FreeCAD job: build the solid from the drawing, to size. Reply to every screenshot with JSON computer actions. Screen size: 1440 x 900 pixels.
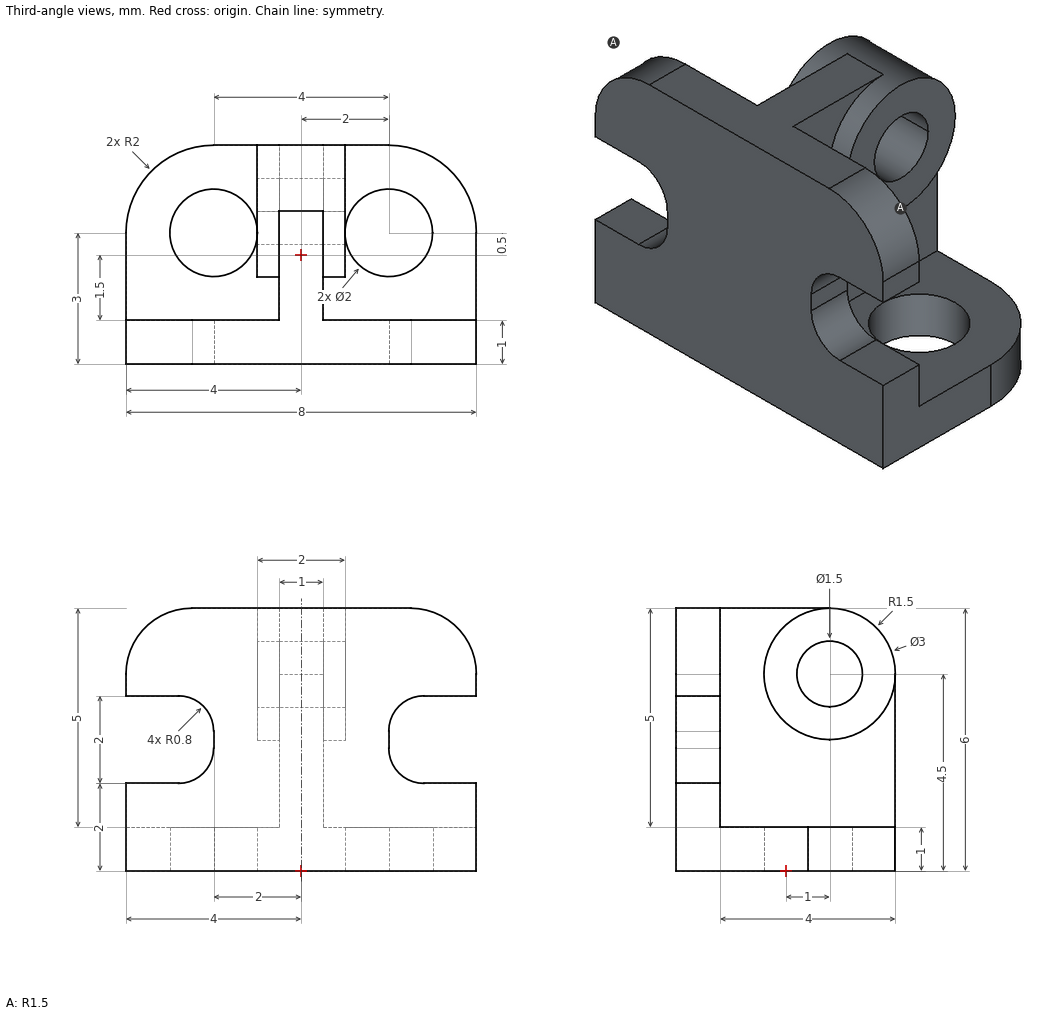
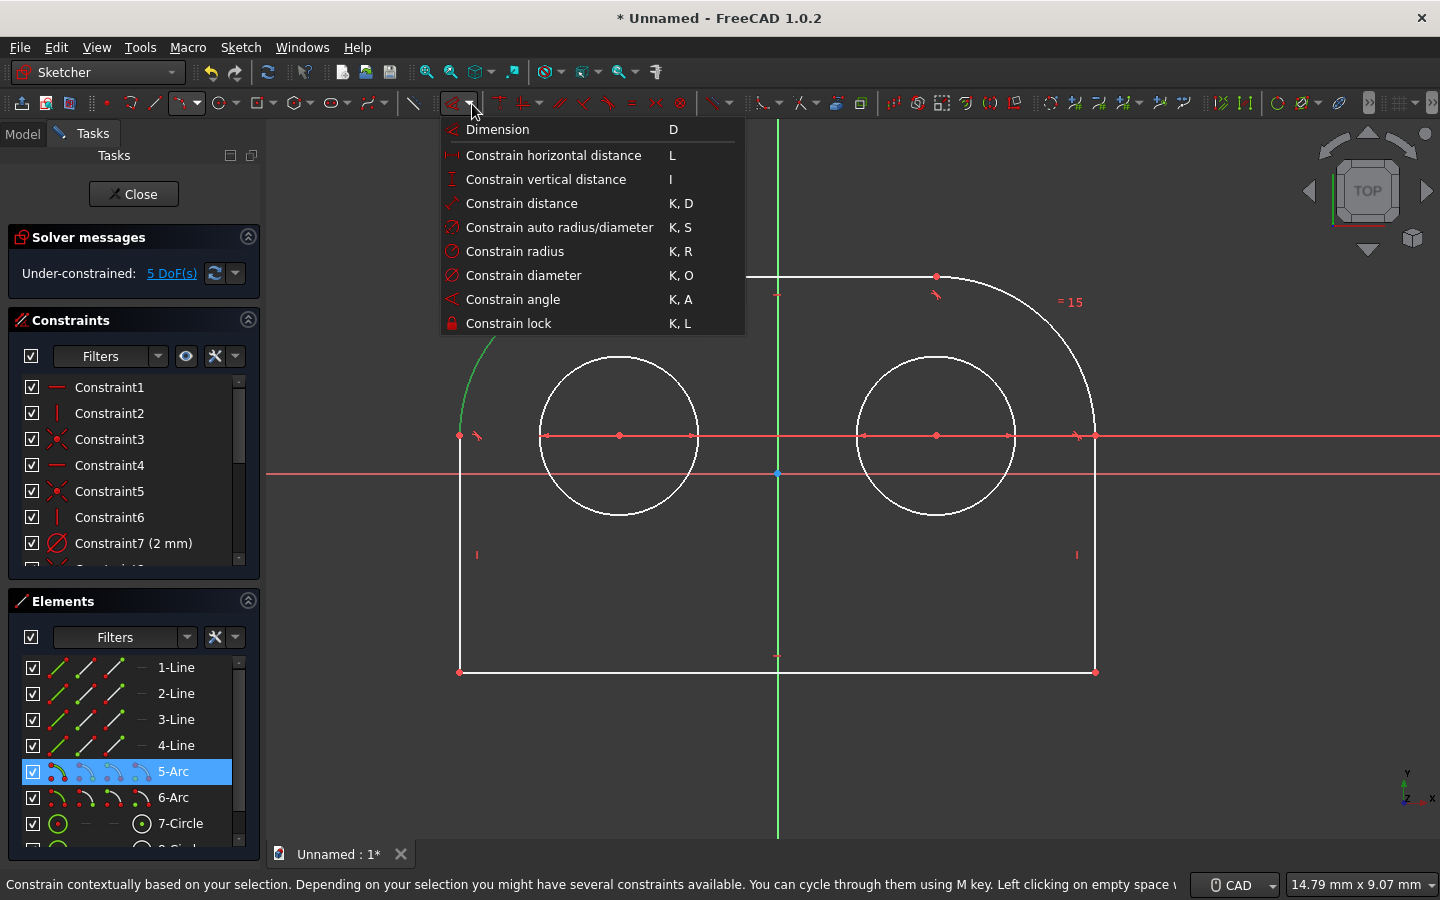
{"action": "left_click", "coordinate": [593, 251]}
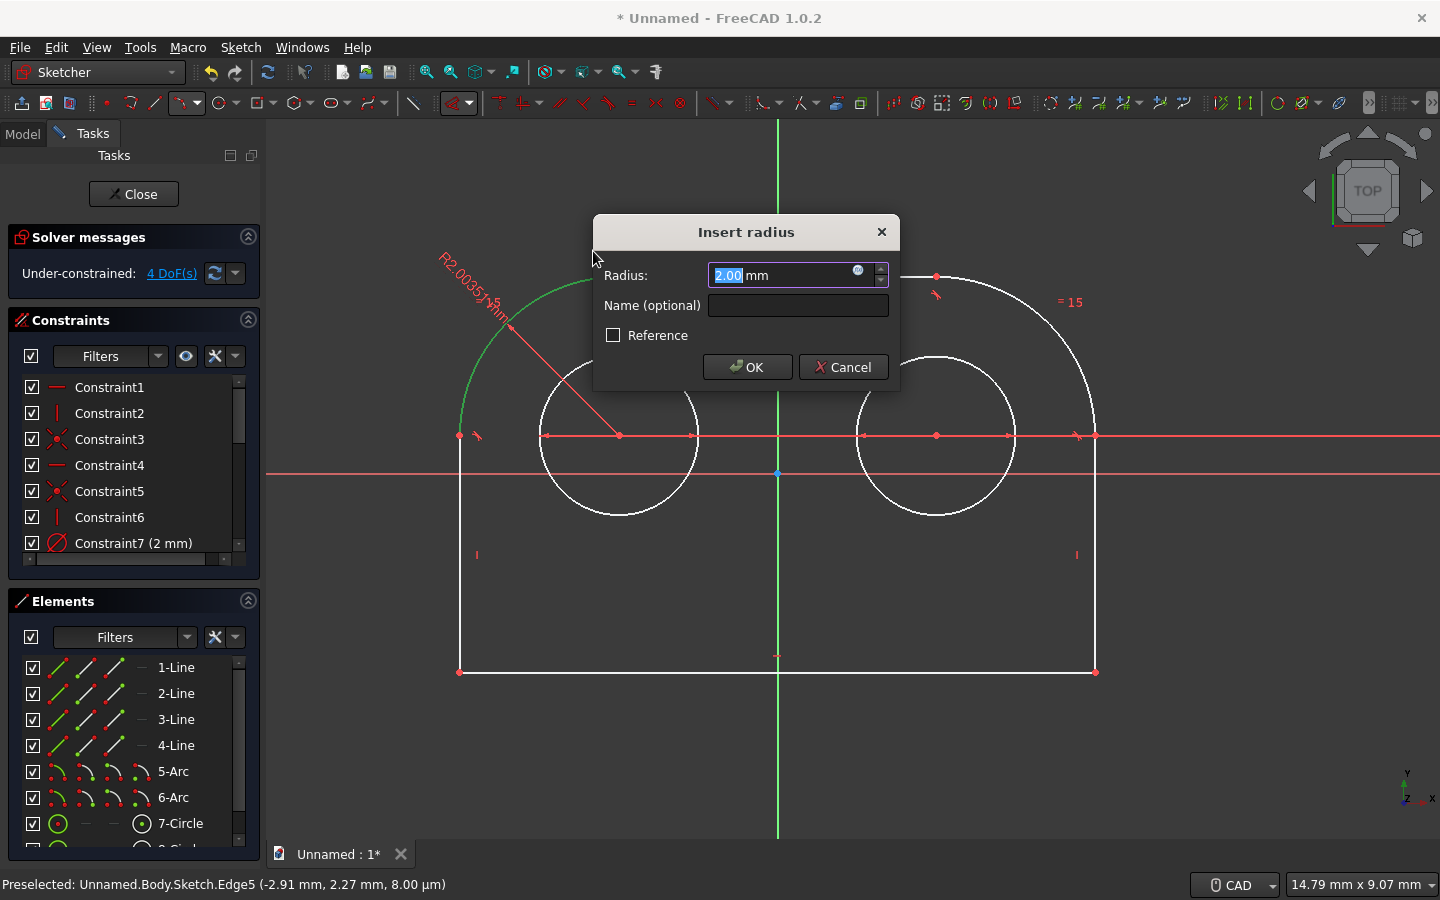
{"action": "type", "text": "2"}
{"action": "key", "text": "Return"}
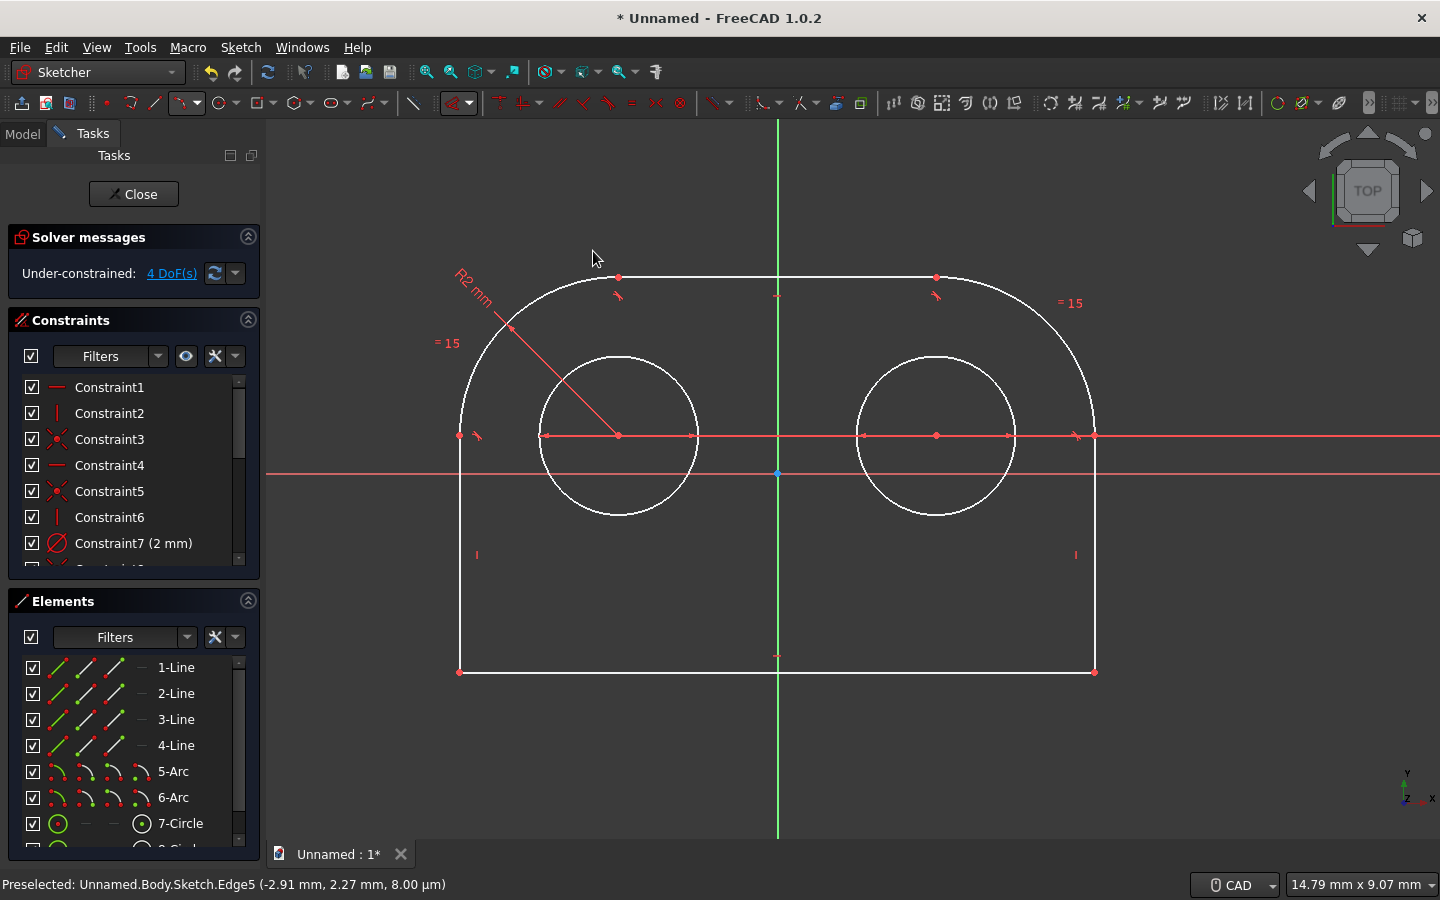
{"action": "left_click", "coordinate": [841, 277]}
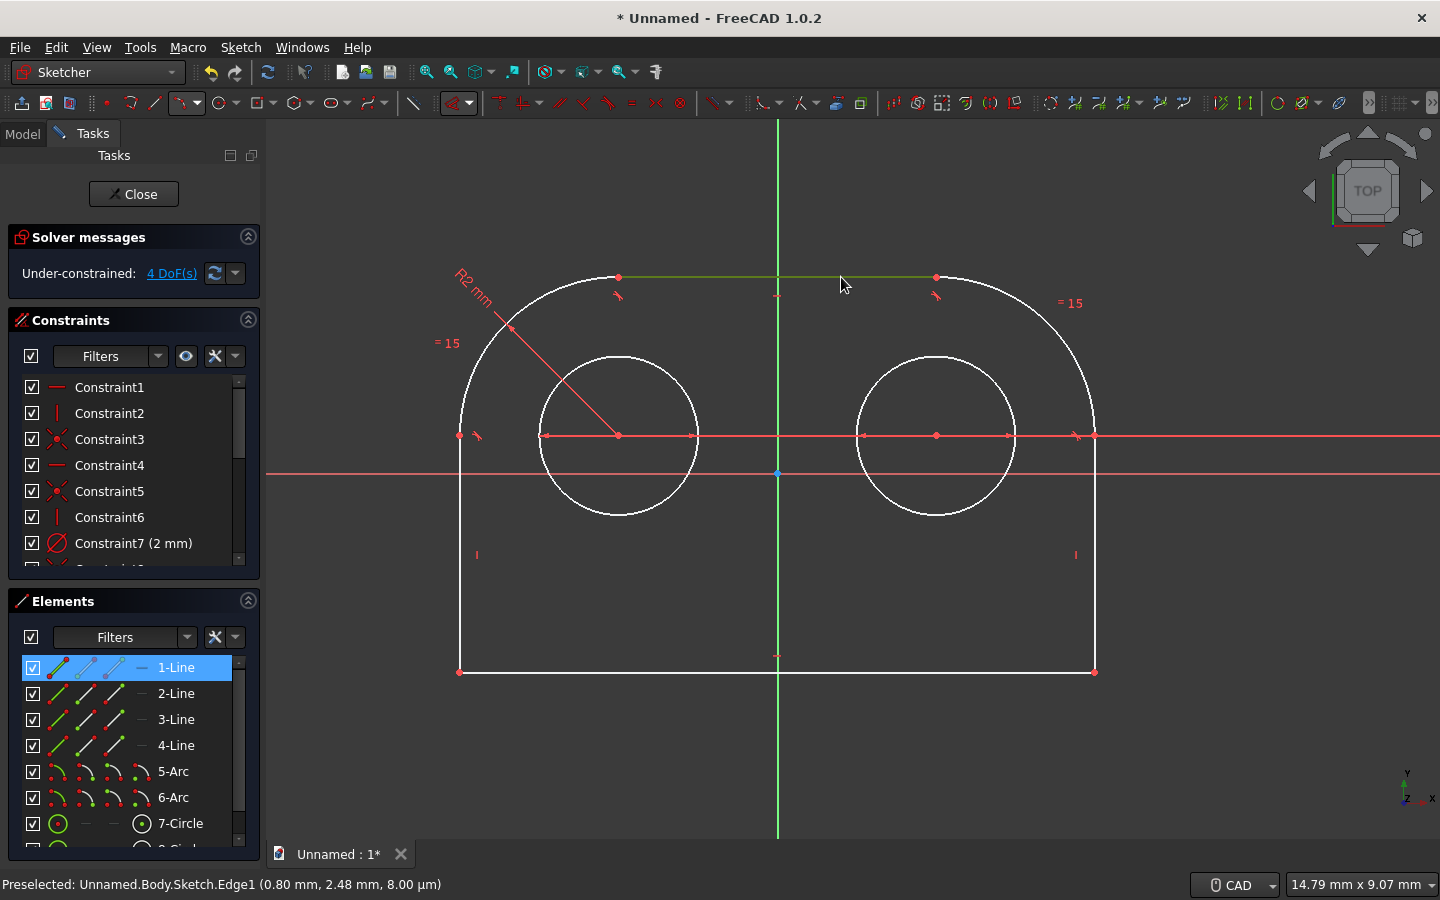
{"action": "left_click", "coordinate": [472, 104]}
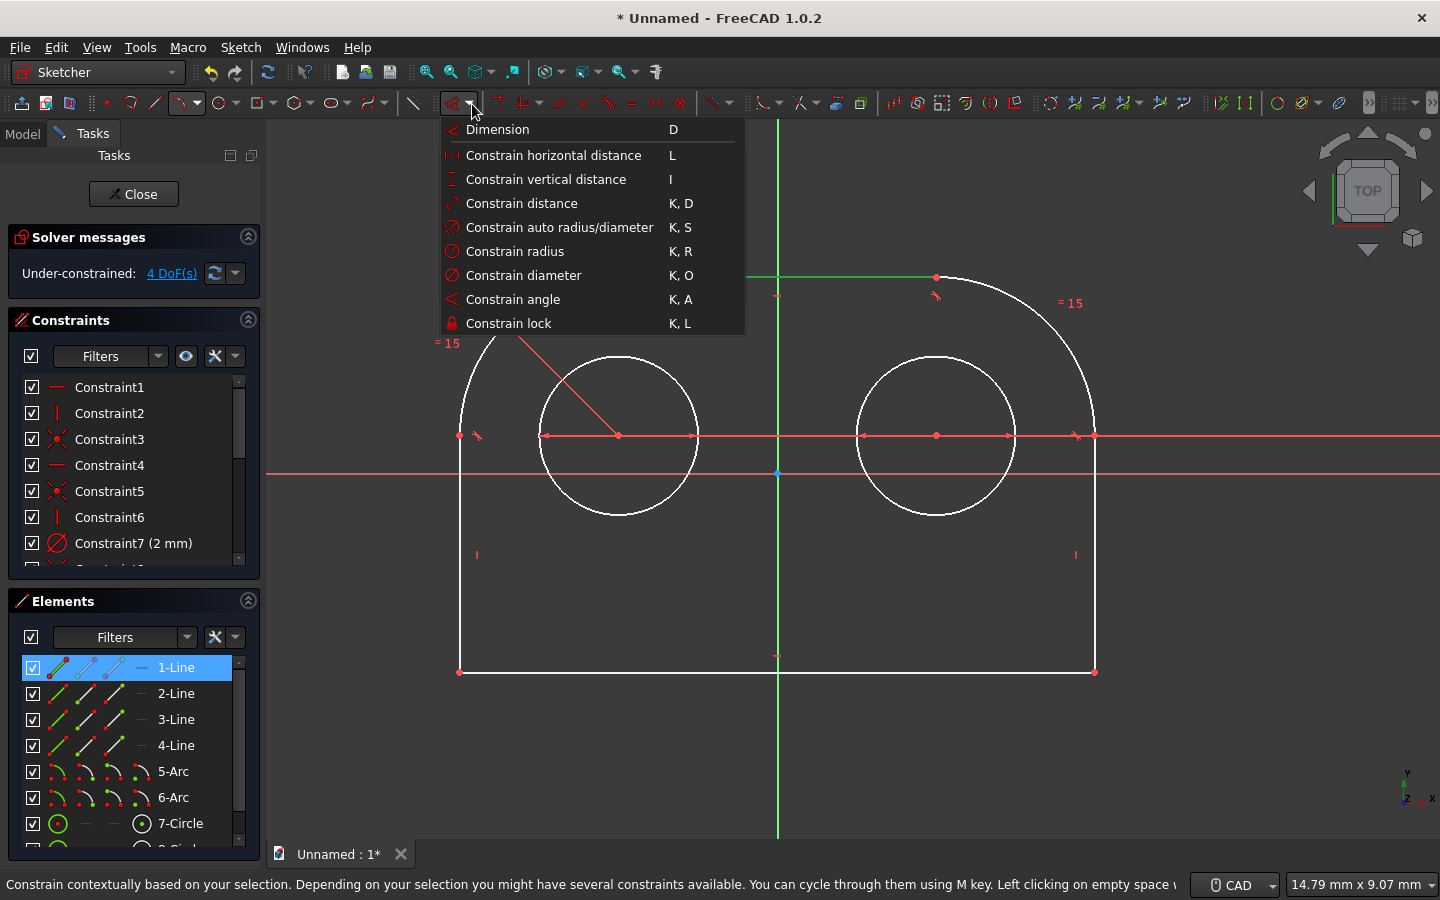
{"action": "left_click", "coordinate": [593, 155]}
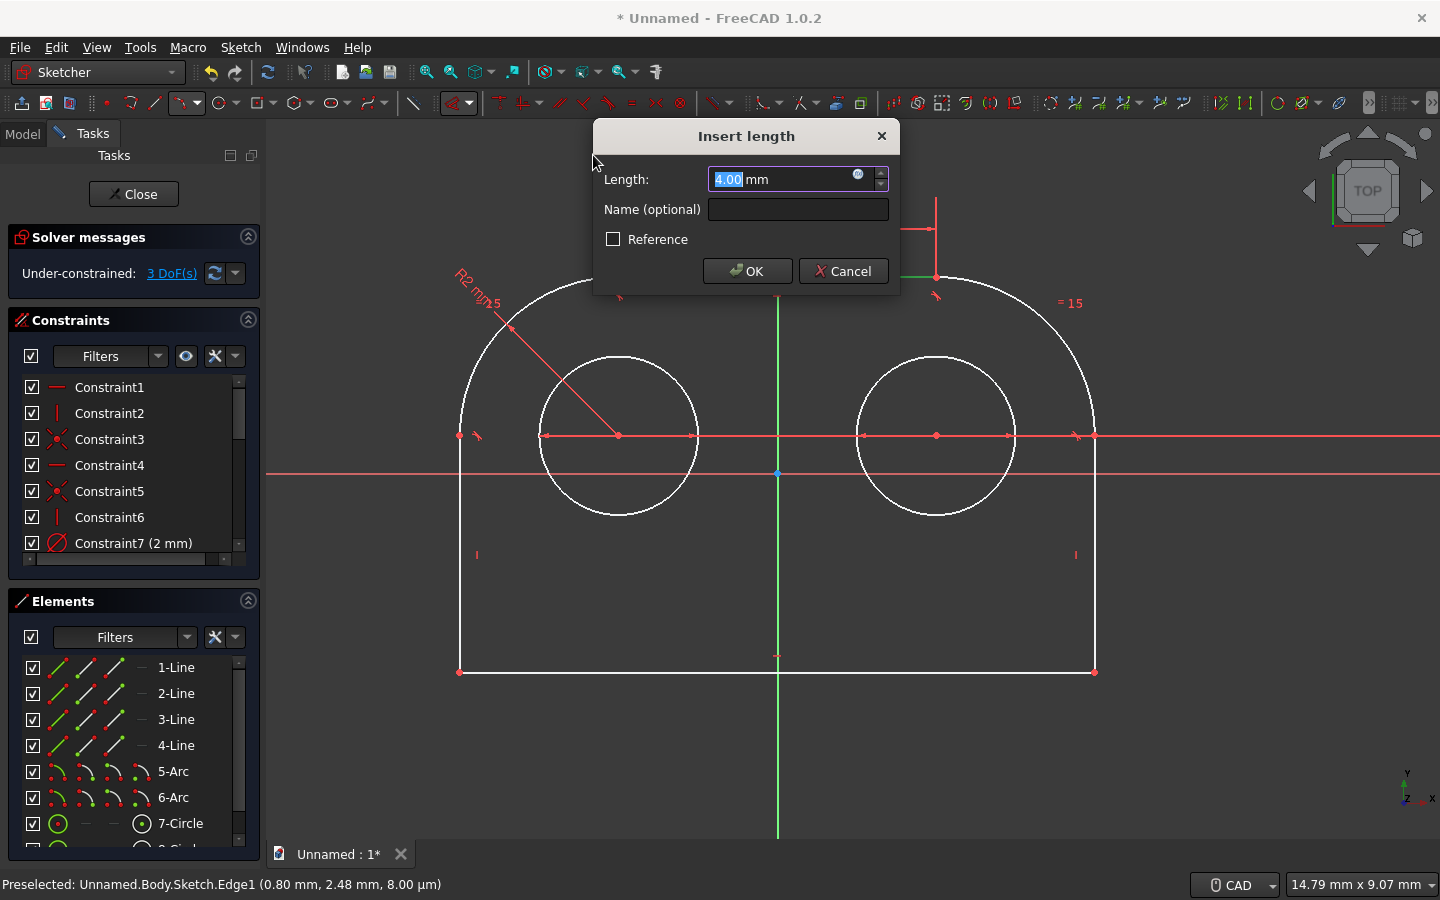
{"action": "type", "text": "4"}
{"action": "key", "text": "Return"}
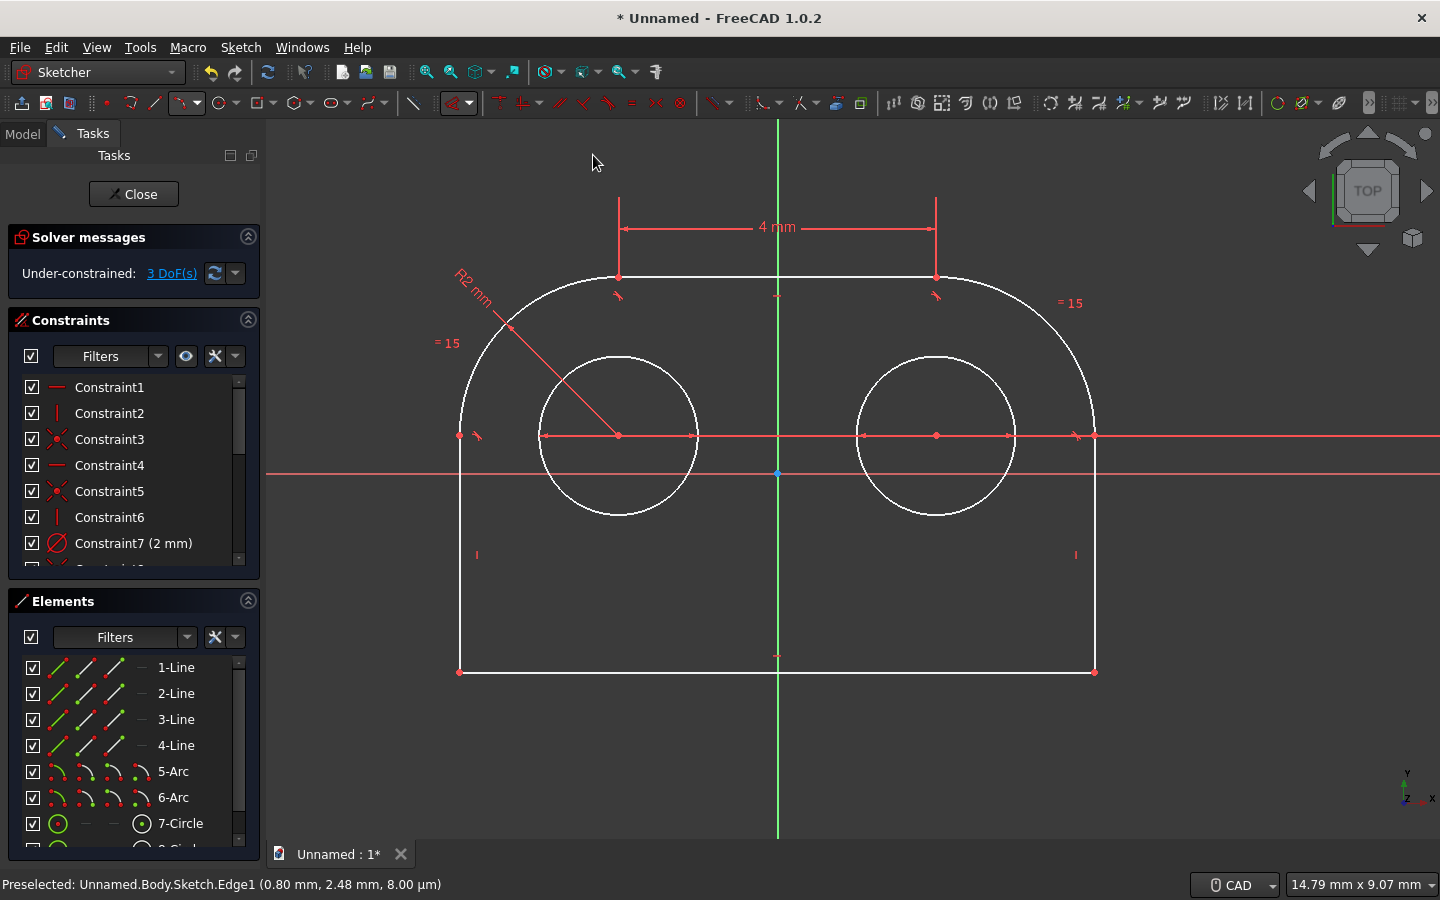
{"action": "left_click", "coordinate": [460, 507]}